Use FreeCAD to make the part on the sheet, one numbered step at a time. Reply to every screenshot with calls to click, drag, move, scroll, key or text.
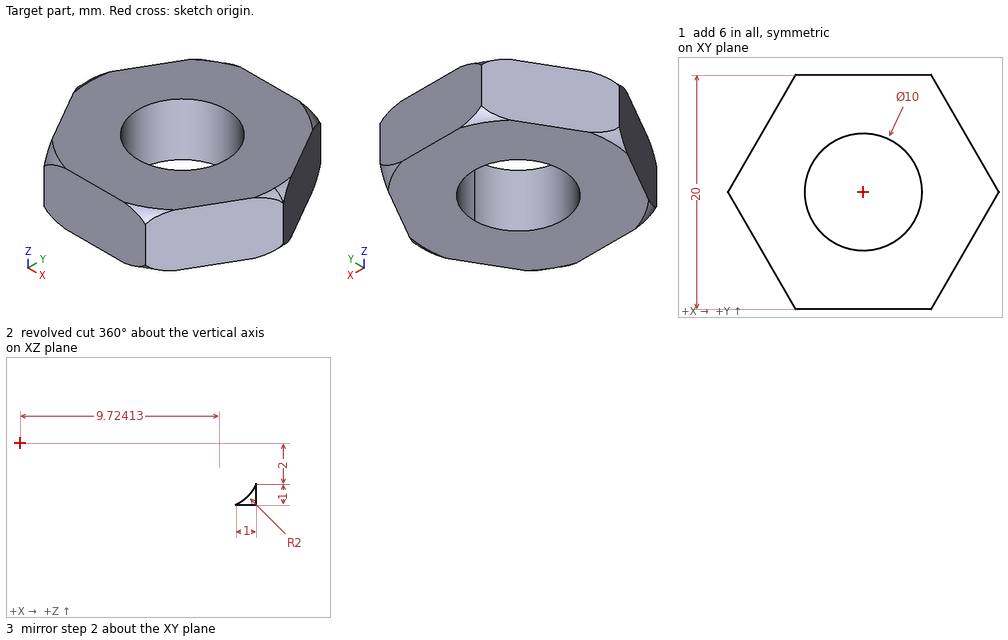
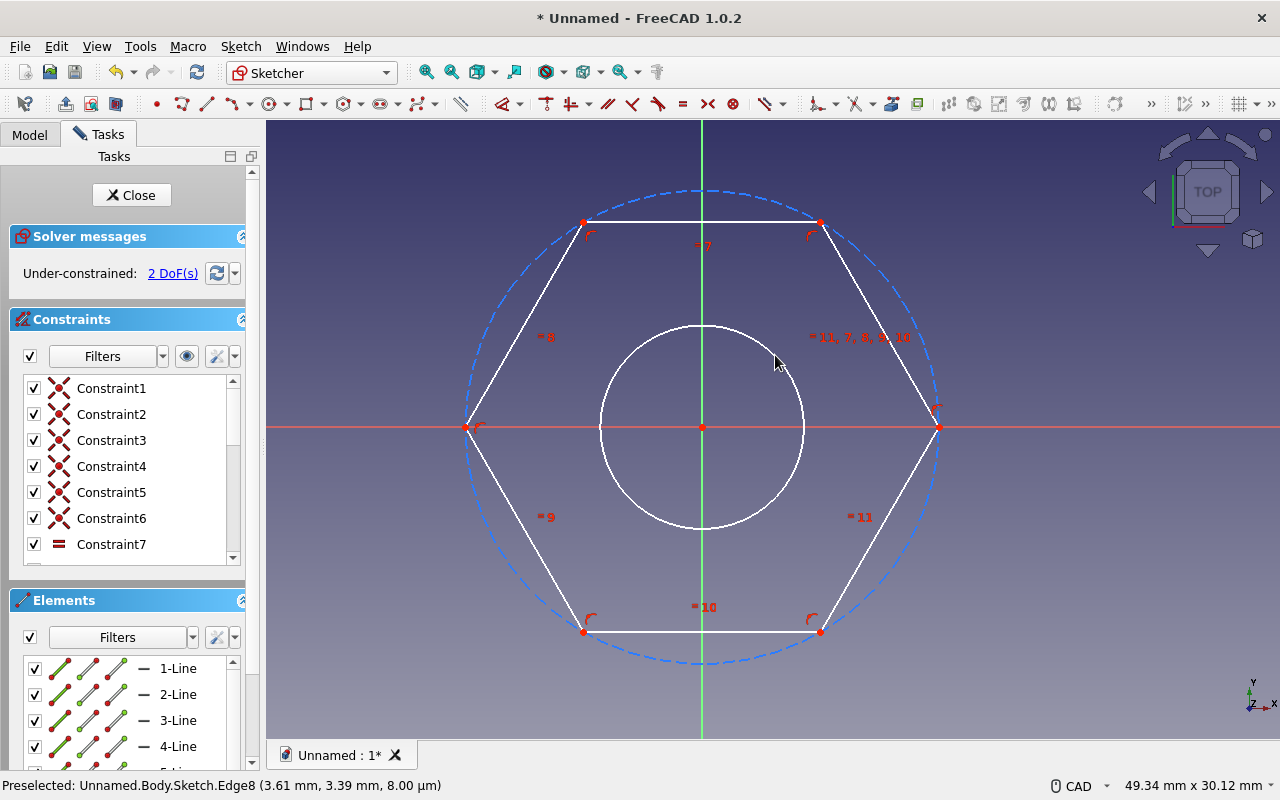
key(d)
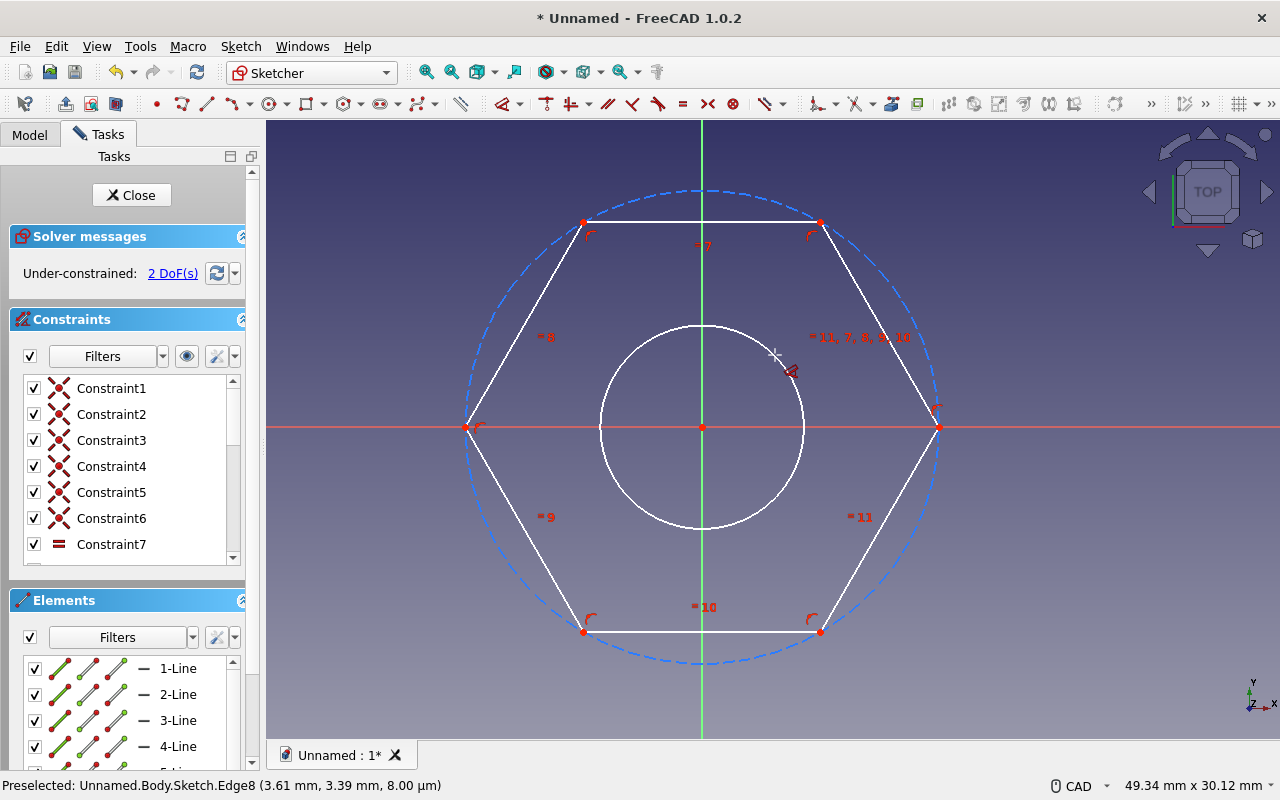
click(774, 355)
click(797, 332)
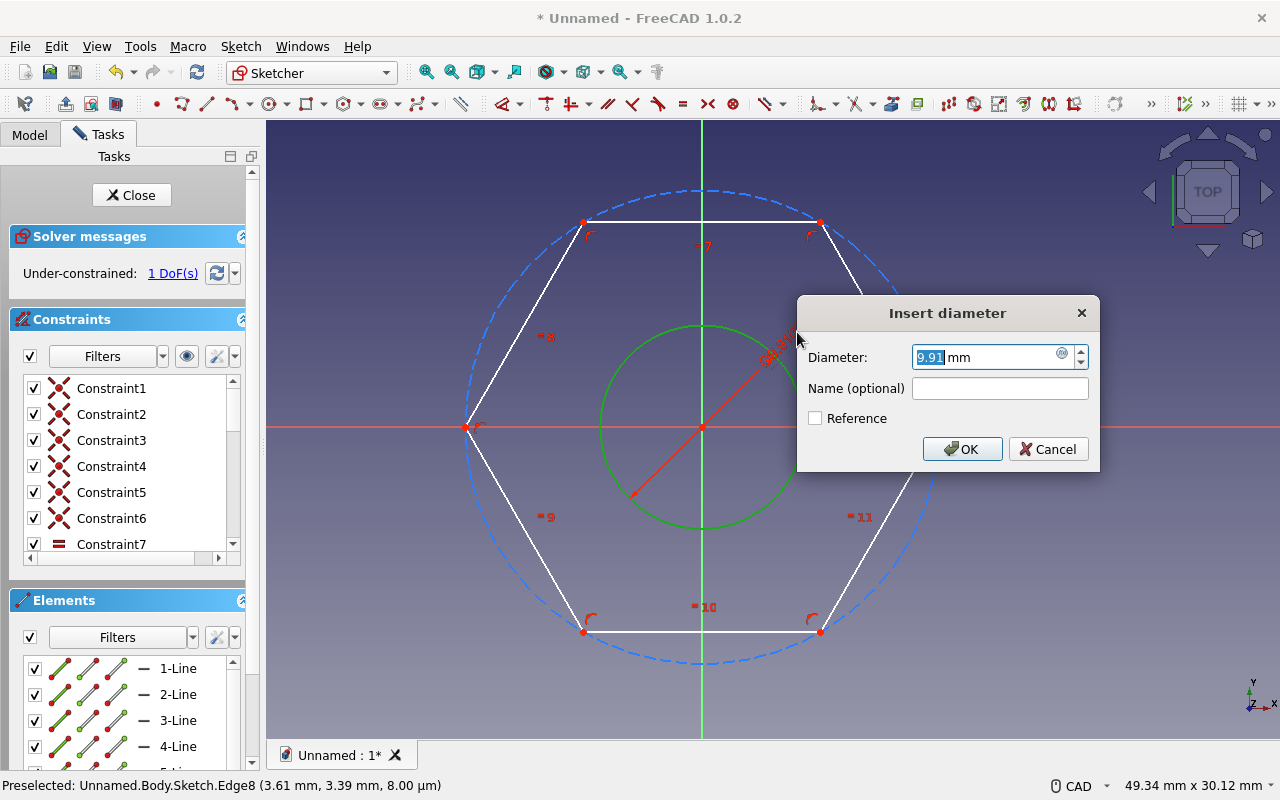
text(10)
key(Return)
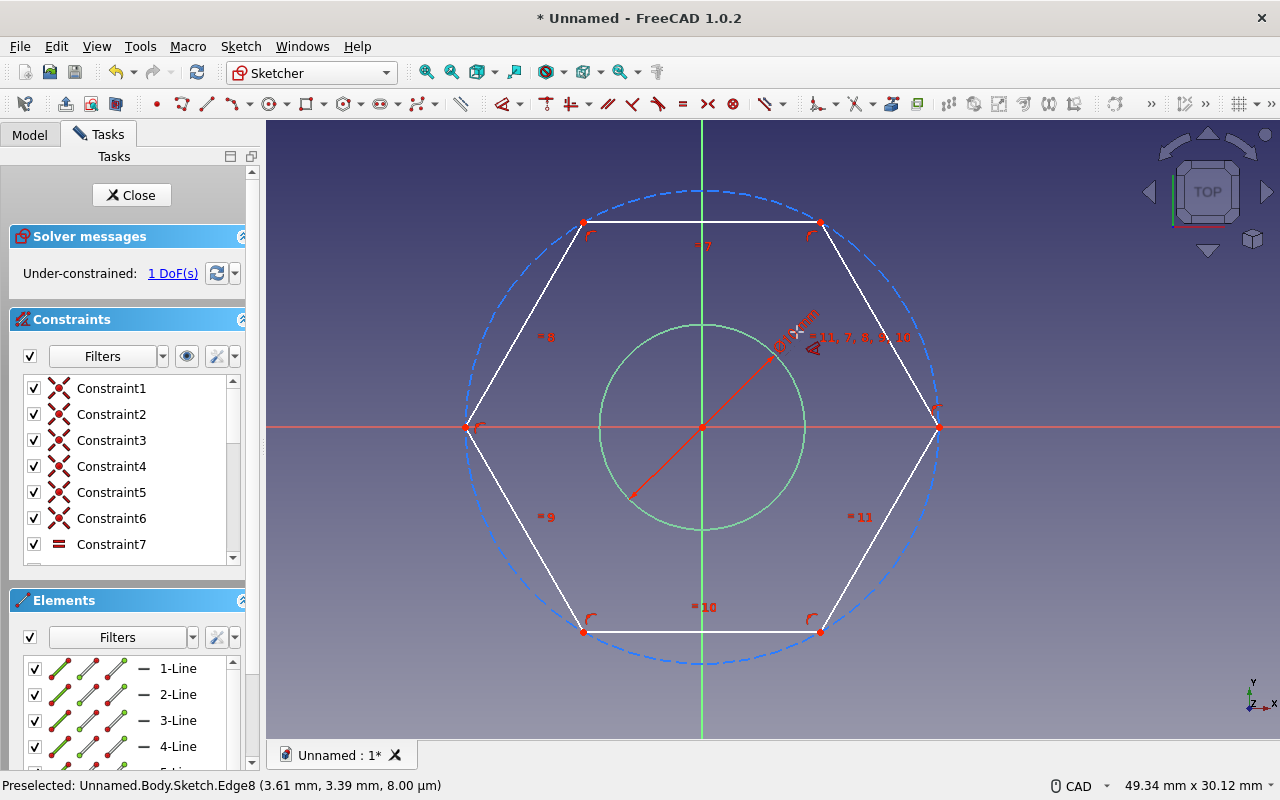
click(584, 632)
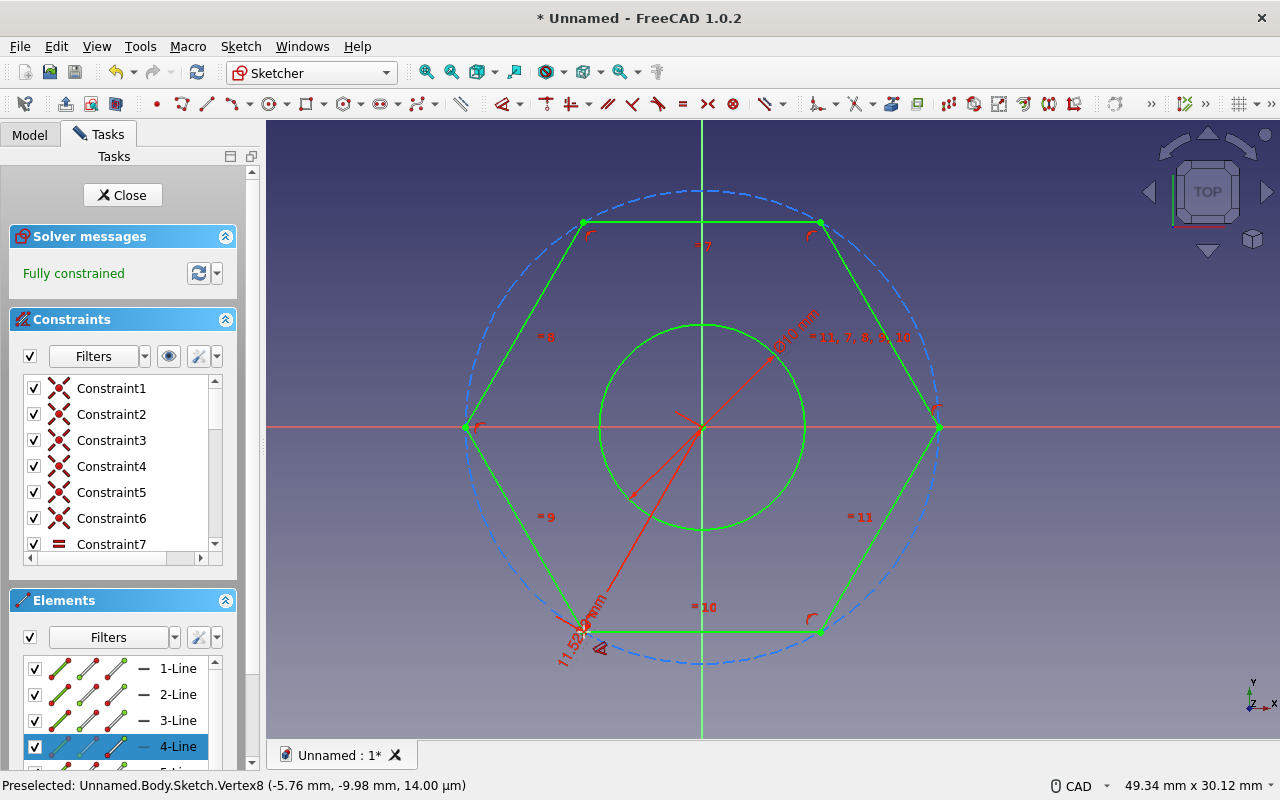
click(821, 222)
click(550, 333)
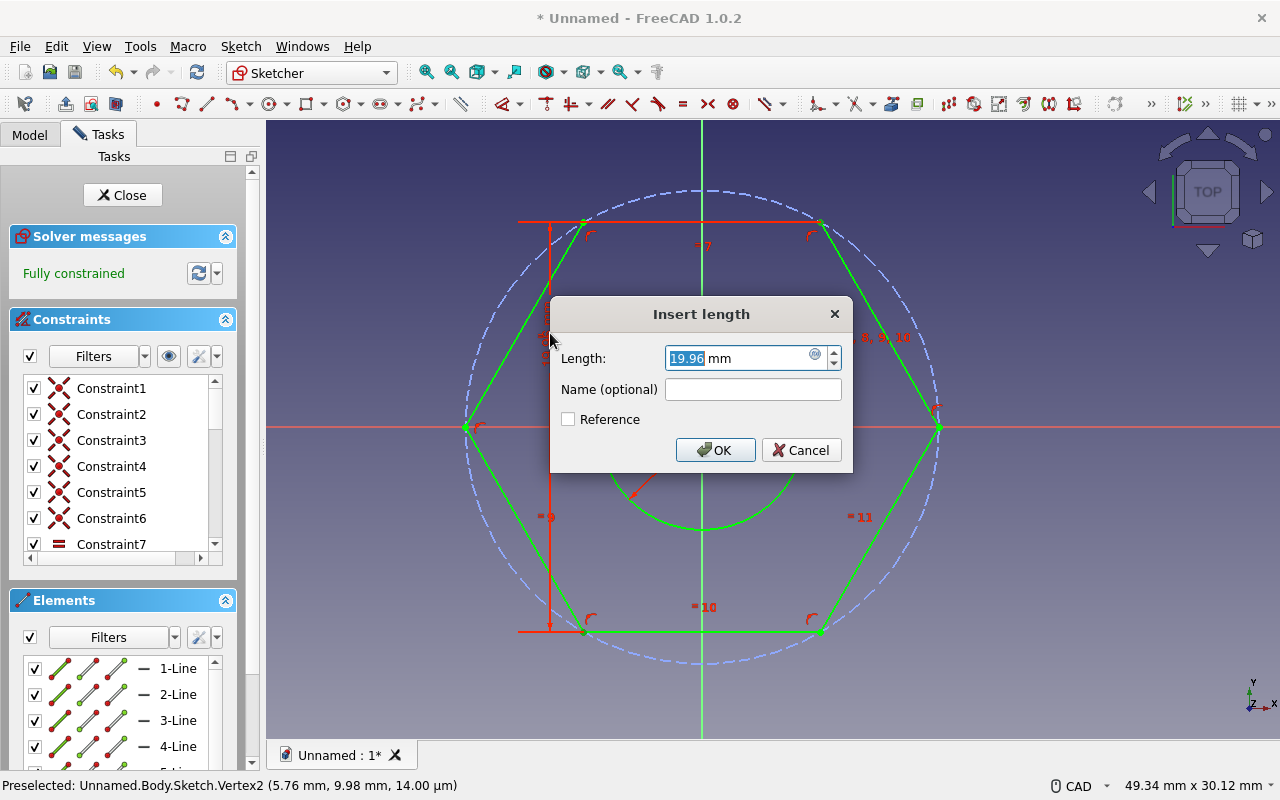
text(20)
key(Return)
key(Escape)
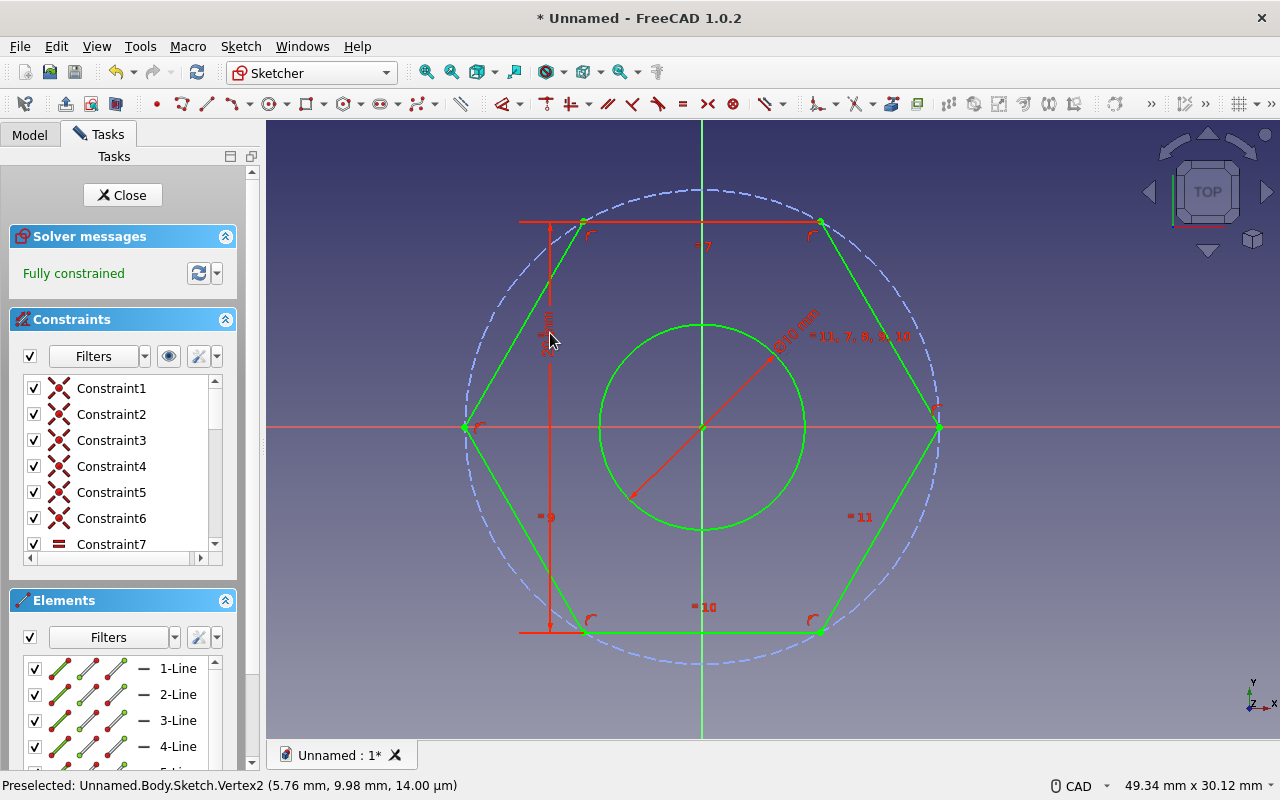
click(123, 195)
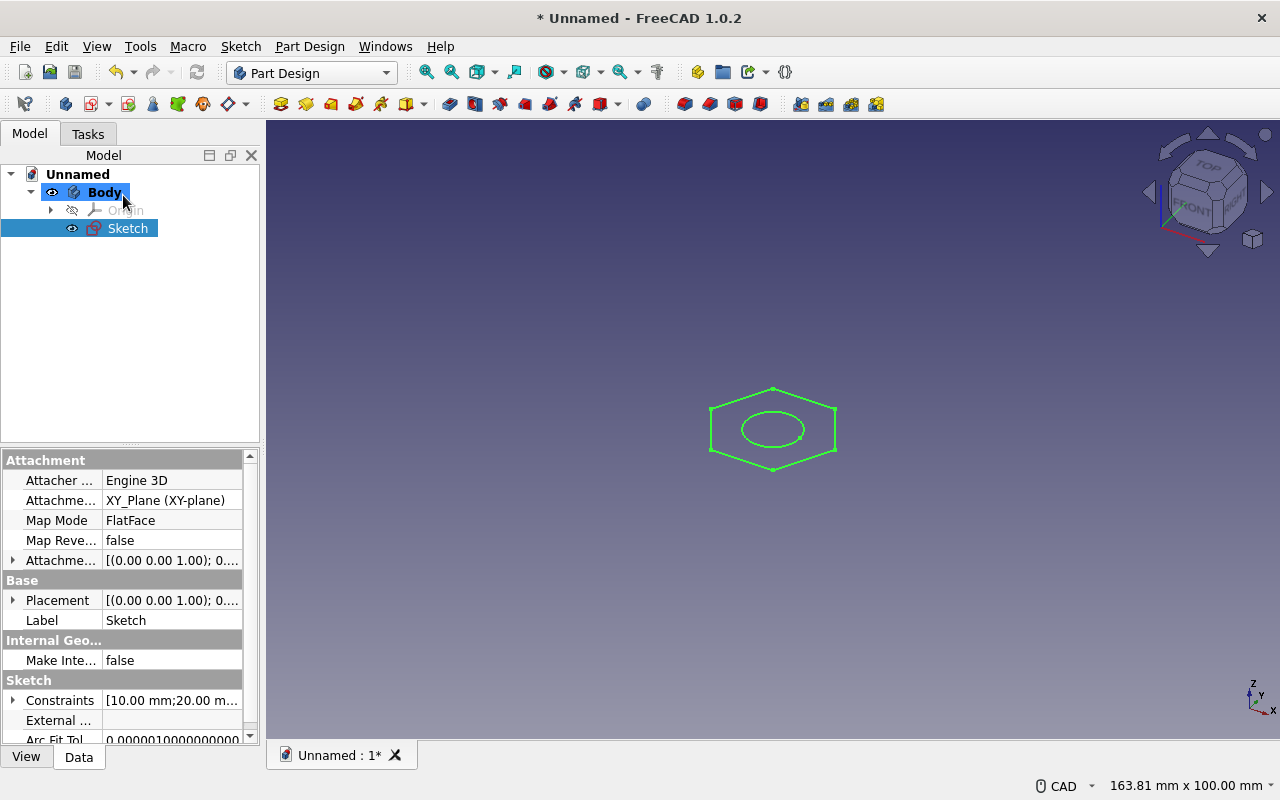
click(281, 104)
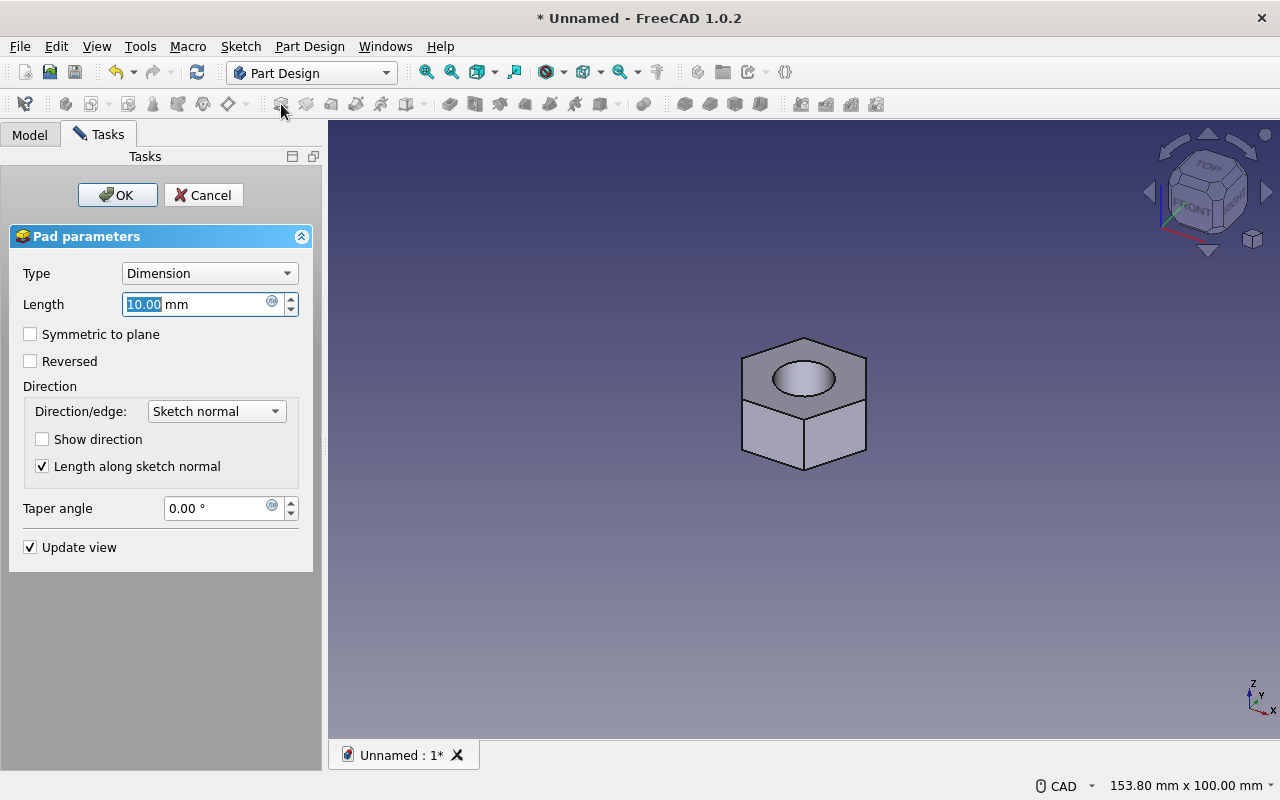
text(6)
key(Tab)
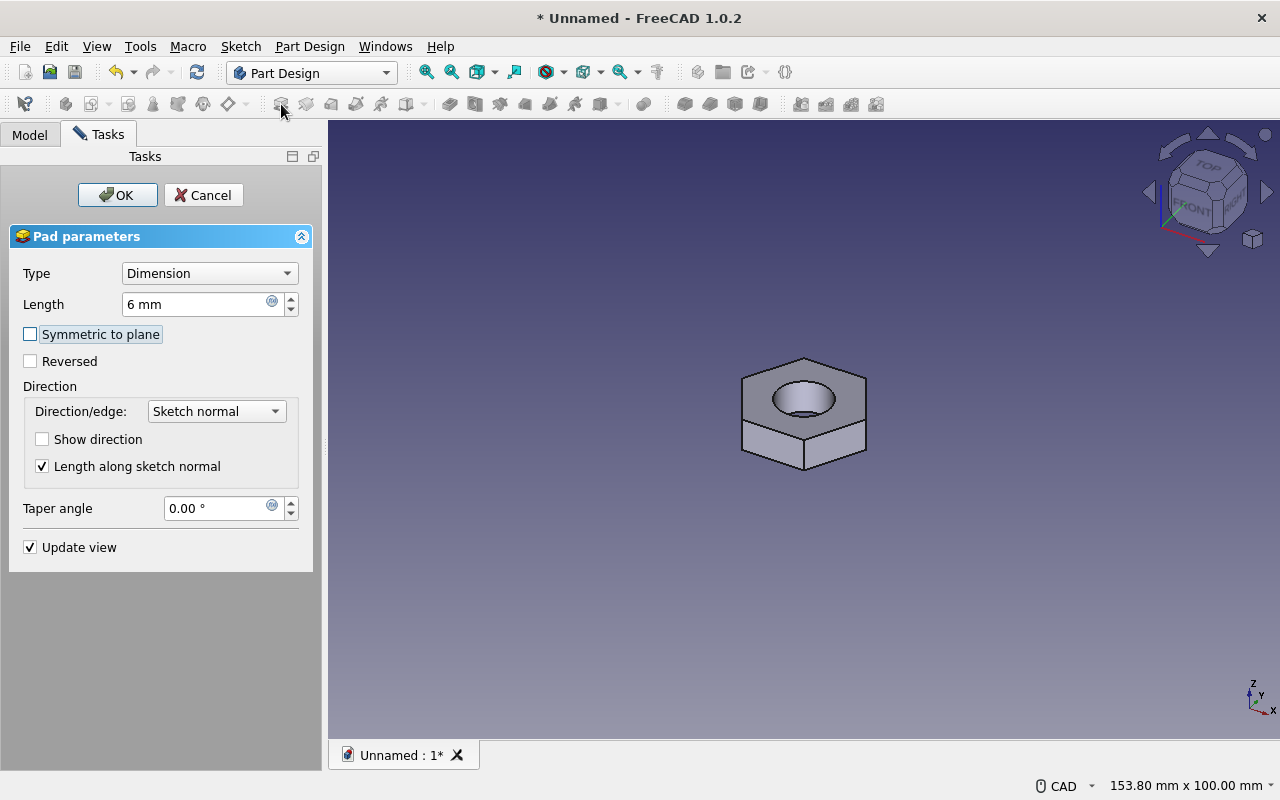
click(31, 334)